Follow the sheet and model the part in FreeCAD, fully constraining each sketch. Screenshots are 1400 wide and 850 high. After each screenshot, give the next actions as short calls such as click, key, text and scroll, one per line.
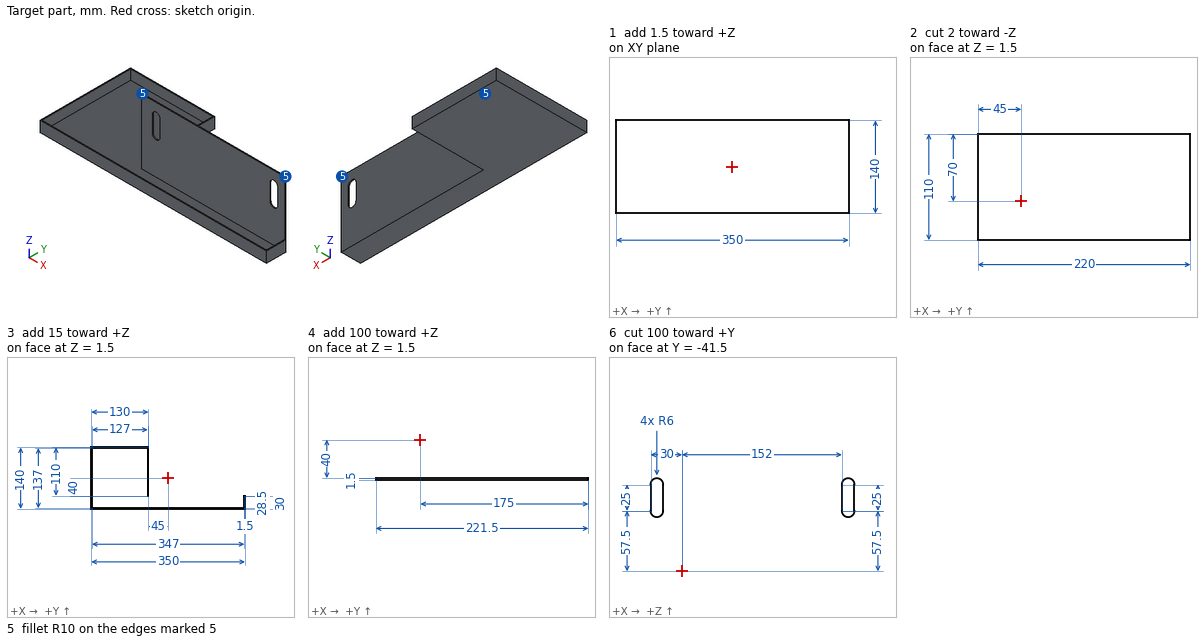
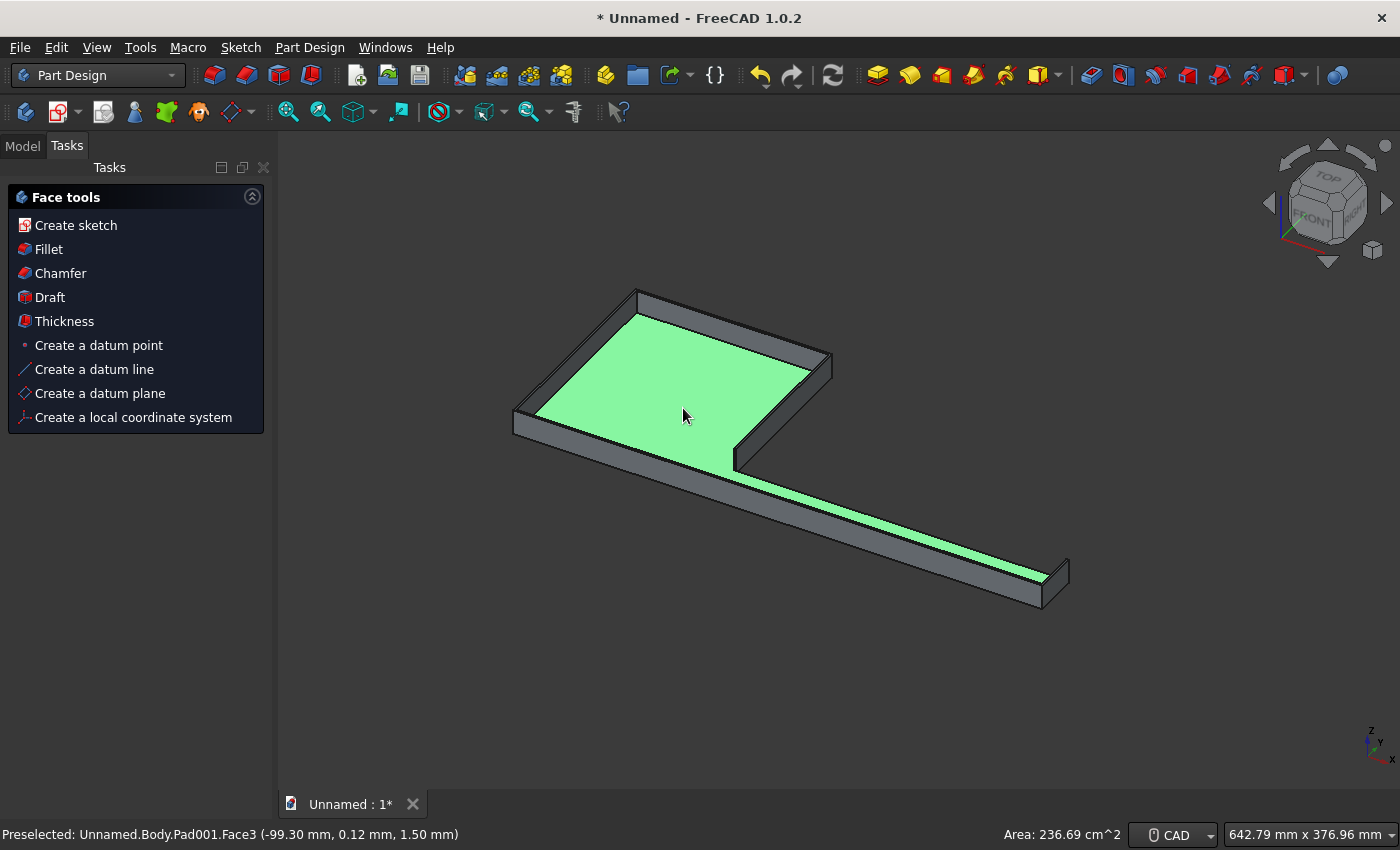
click(58, 112)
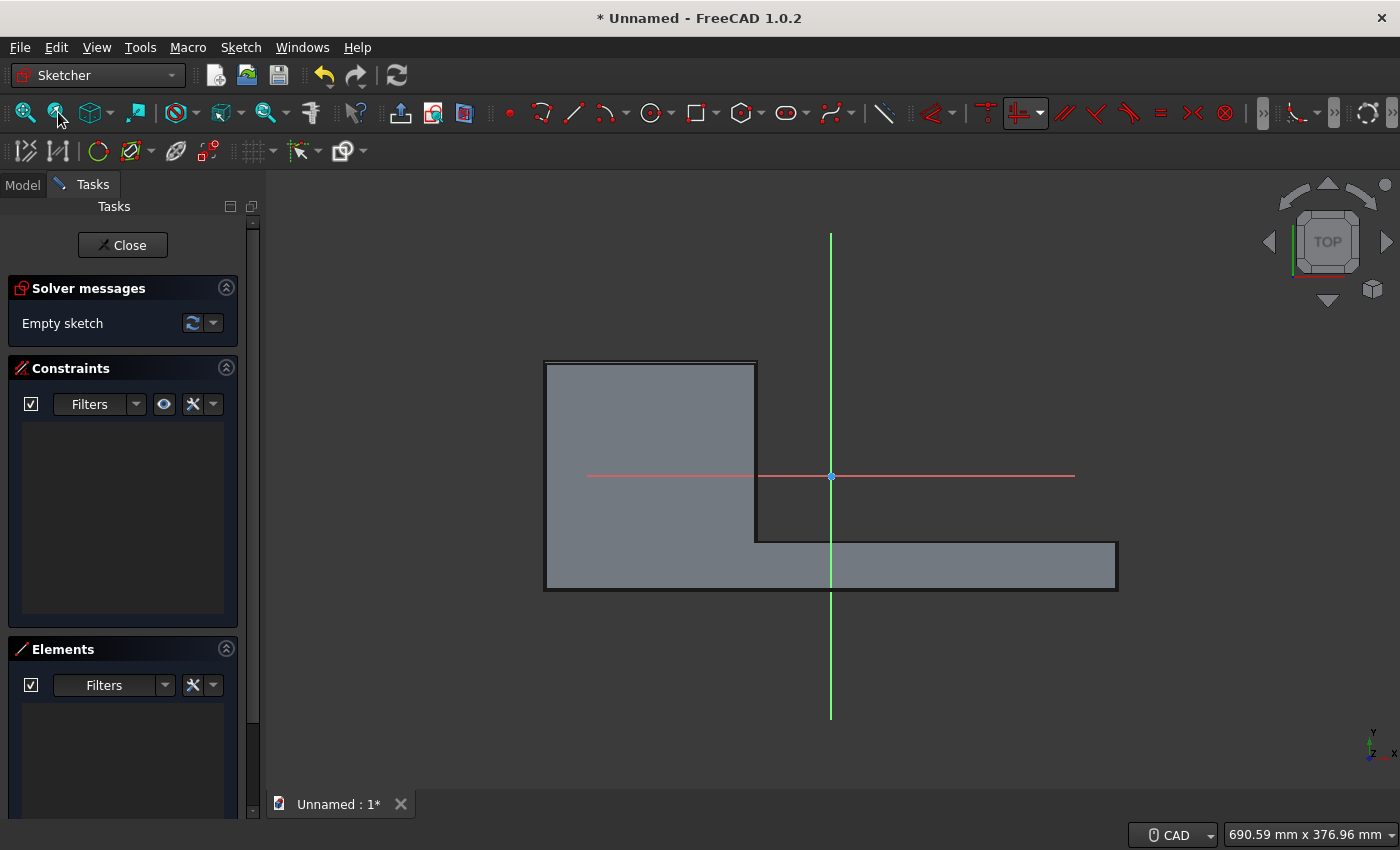
scroll(1146, 548, up, 3)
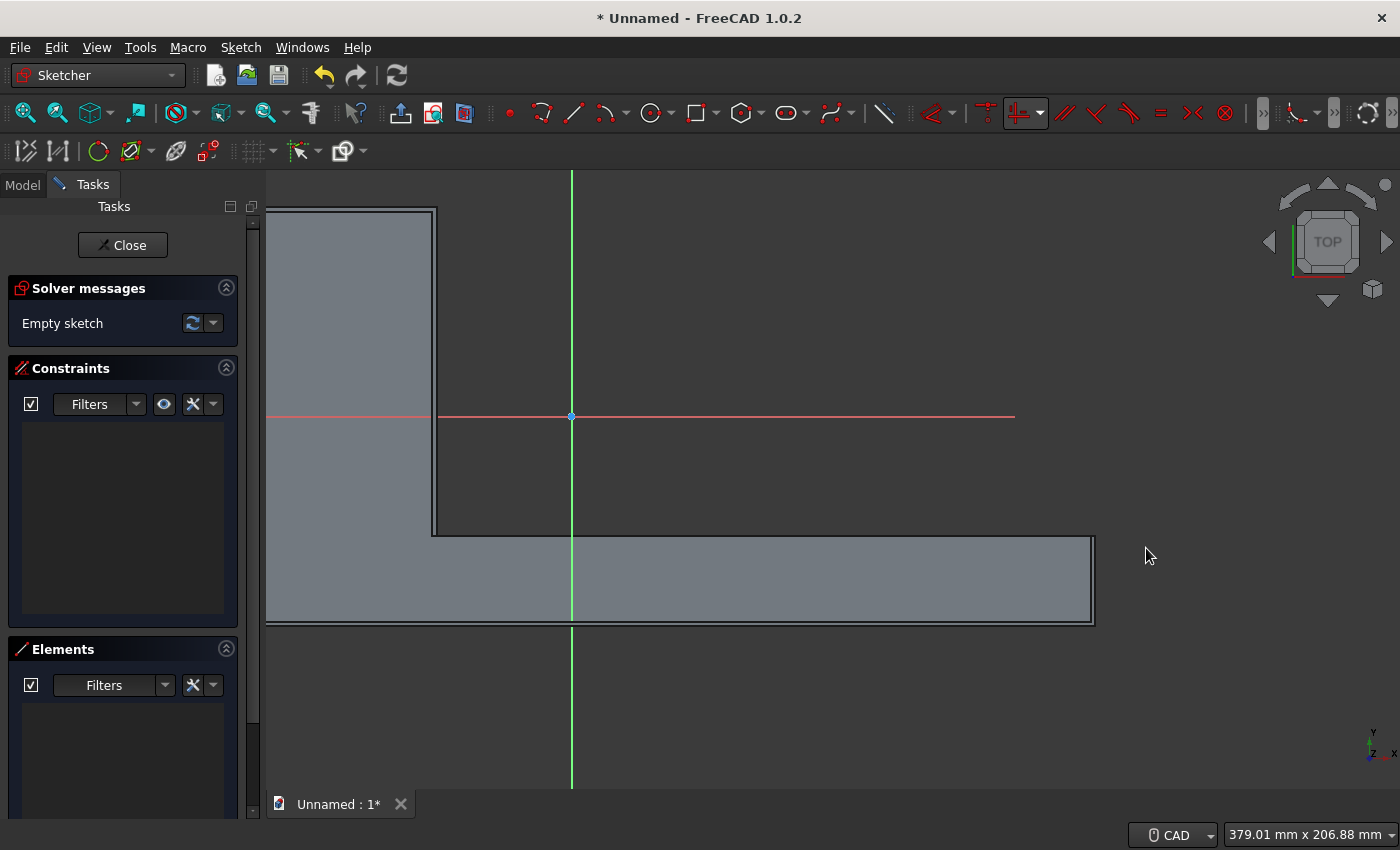
click(696, 114)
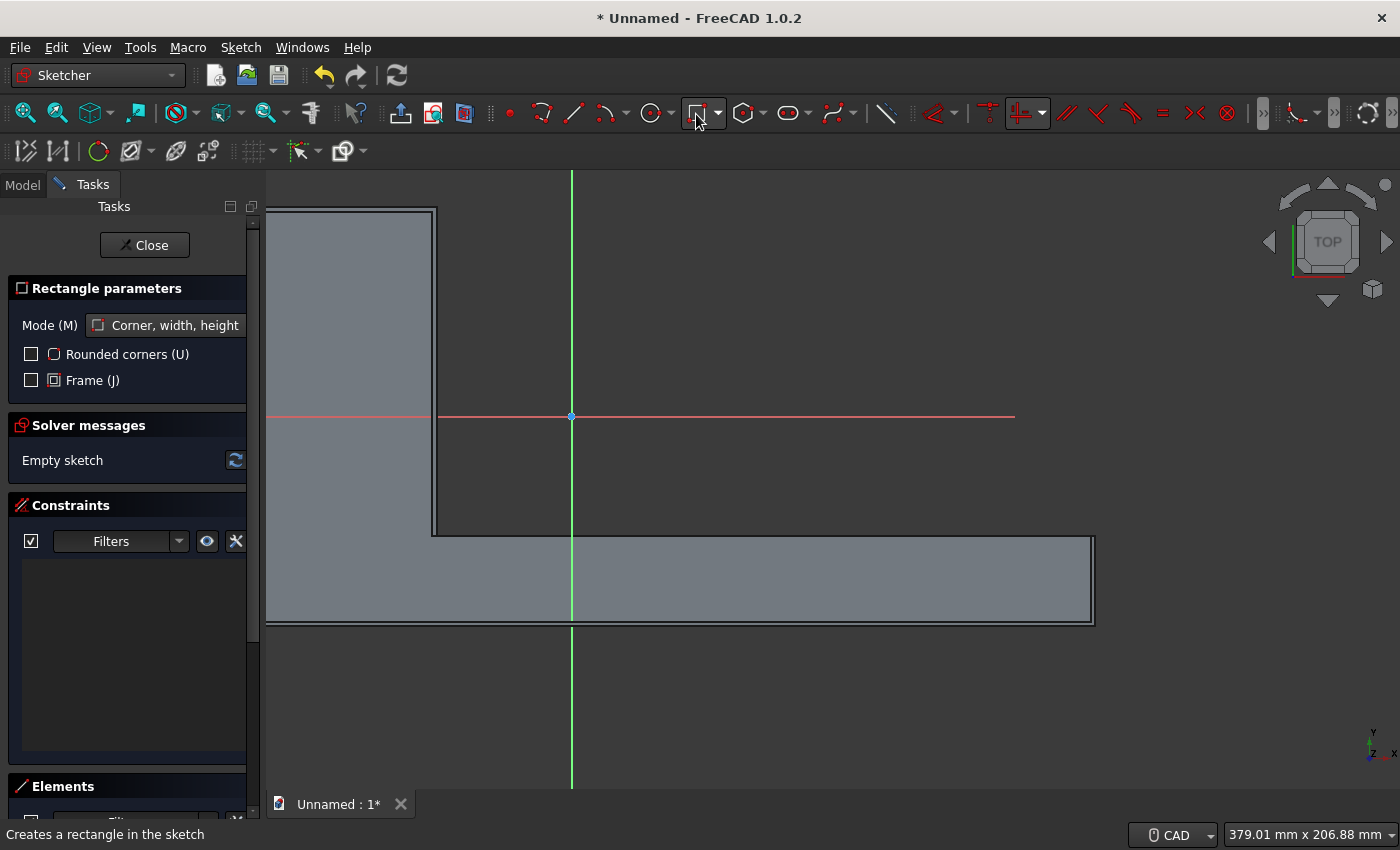
scroll(432, 536, up, 7)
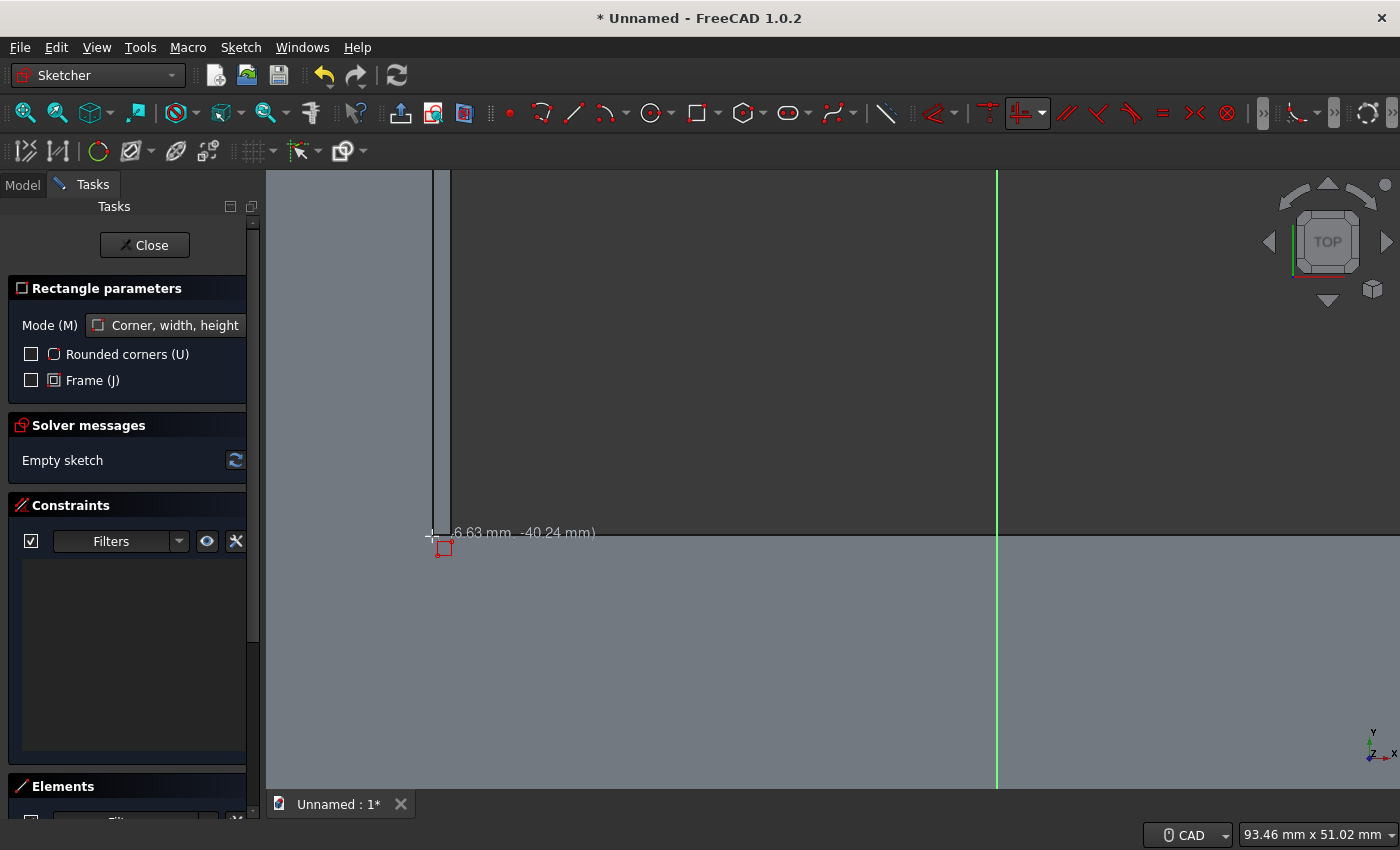
scroll(433, 538, down, 7)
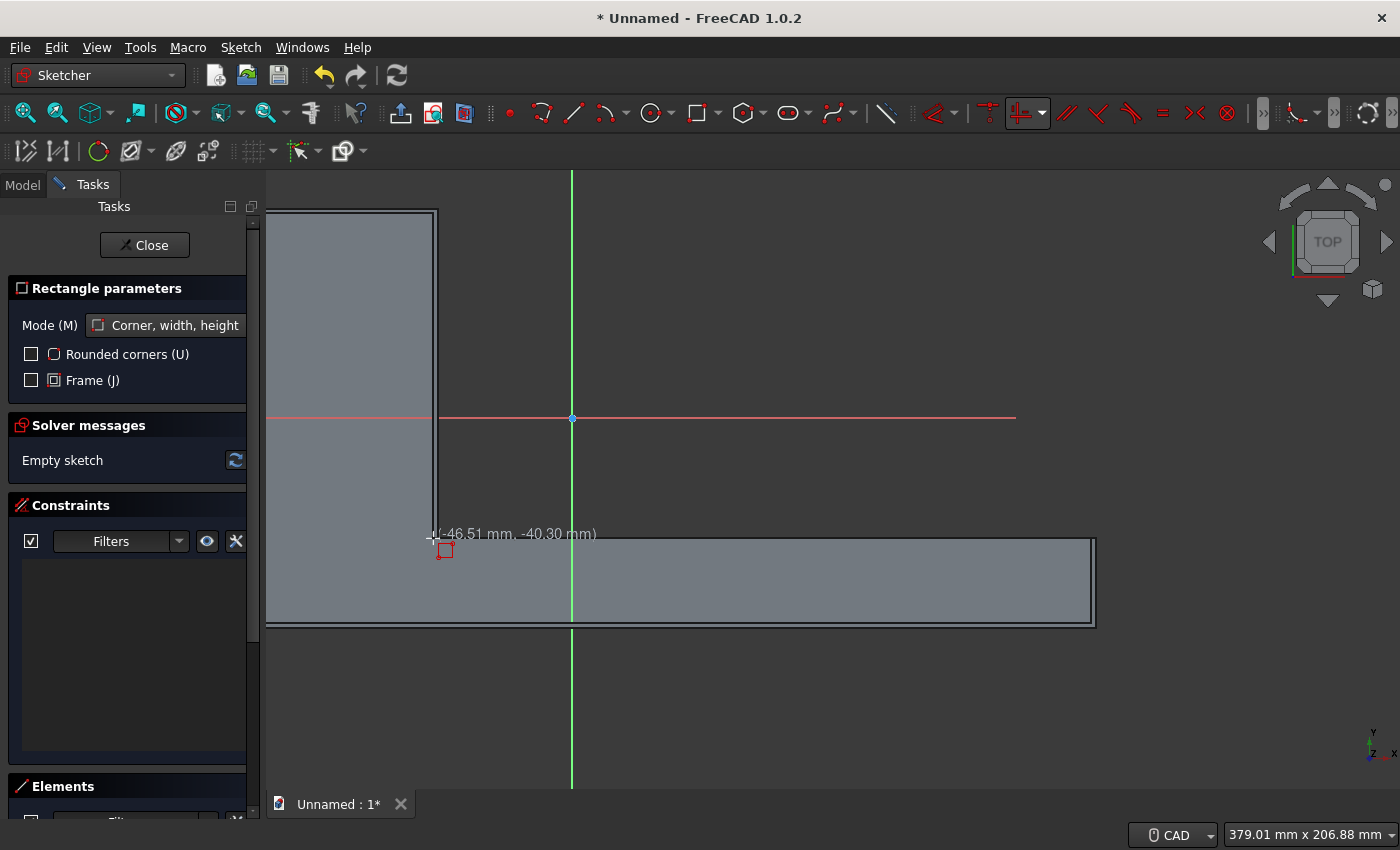
click(433, 538)
click(1096, 542)
key(Escape)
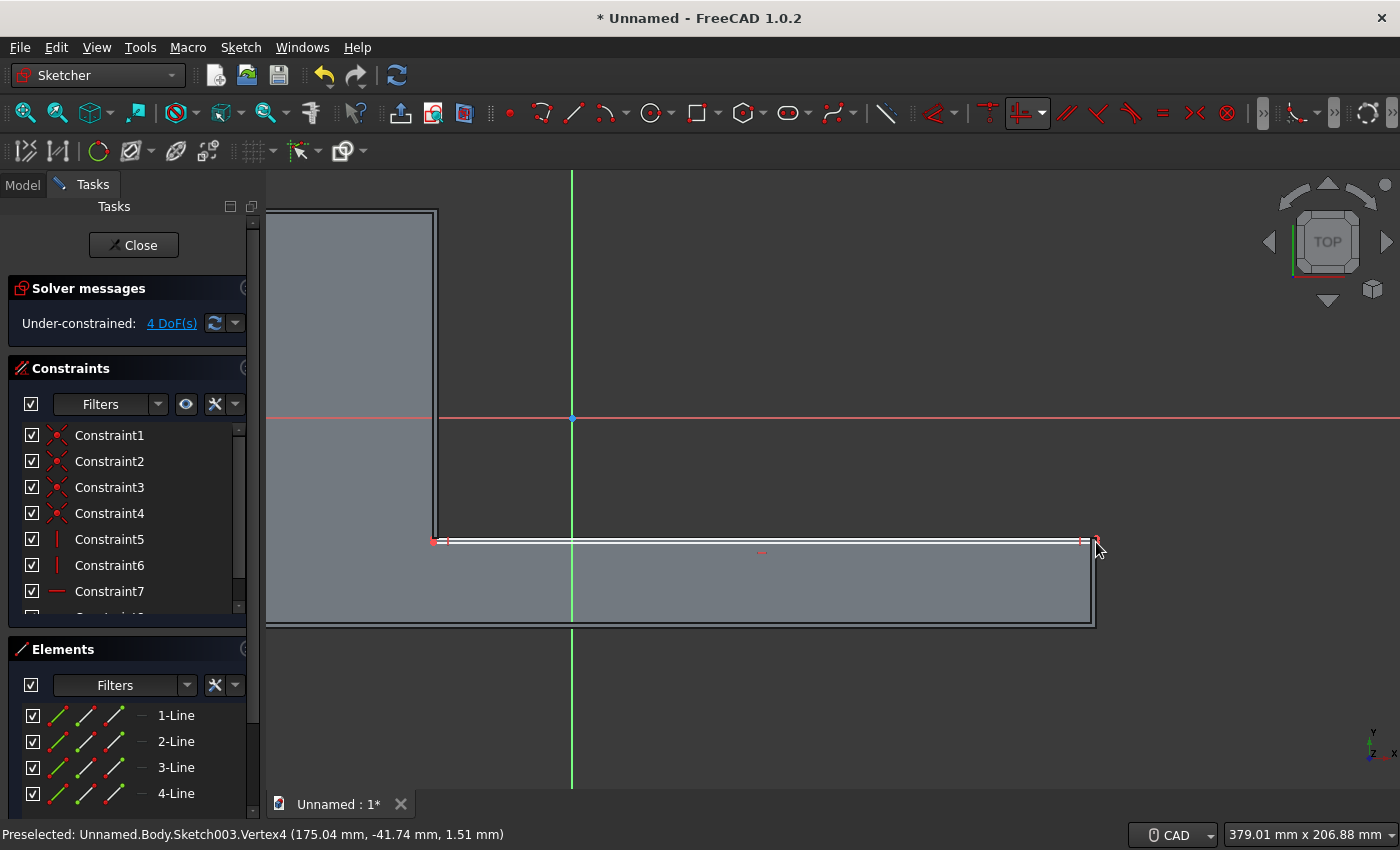
click(934, 114)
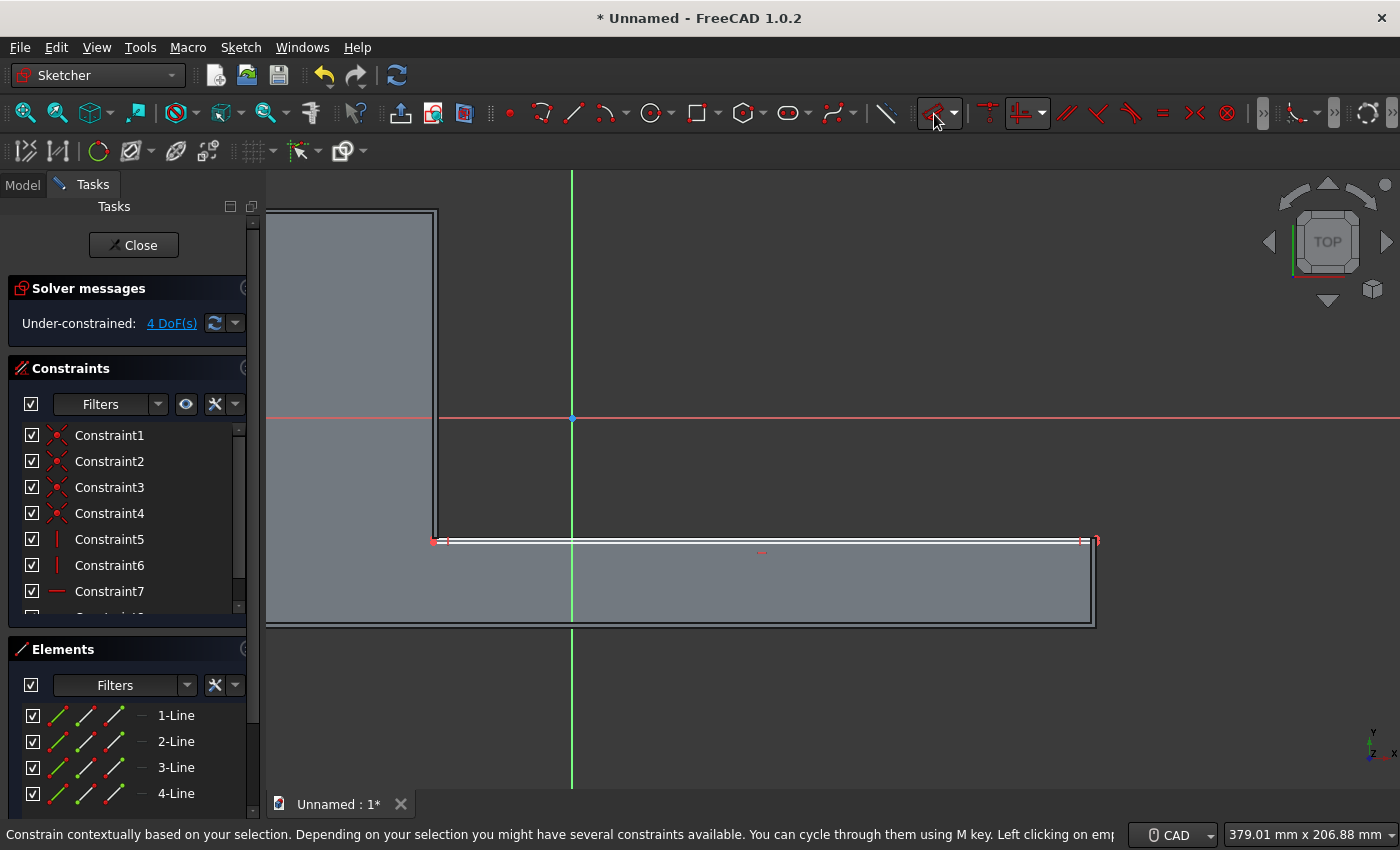
scroll(433, 541, up, 11)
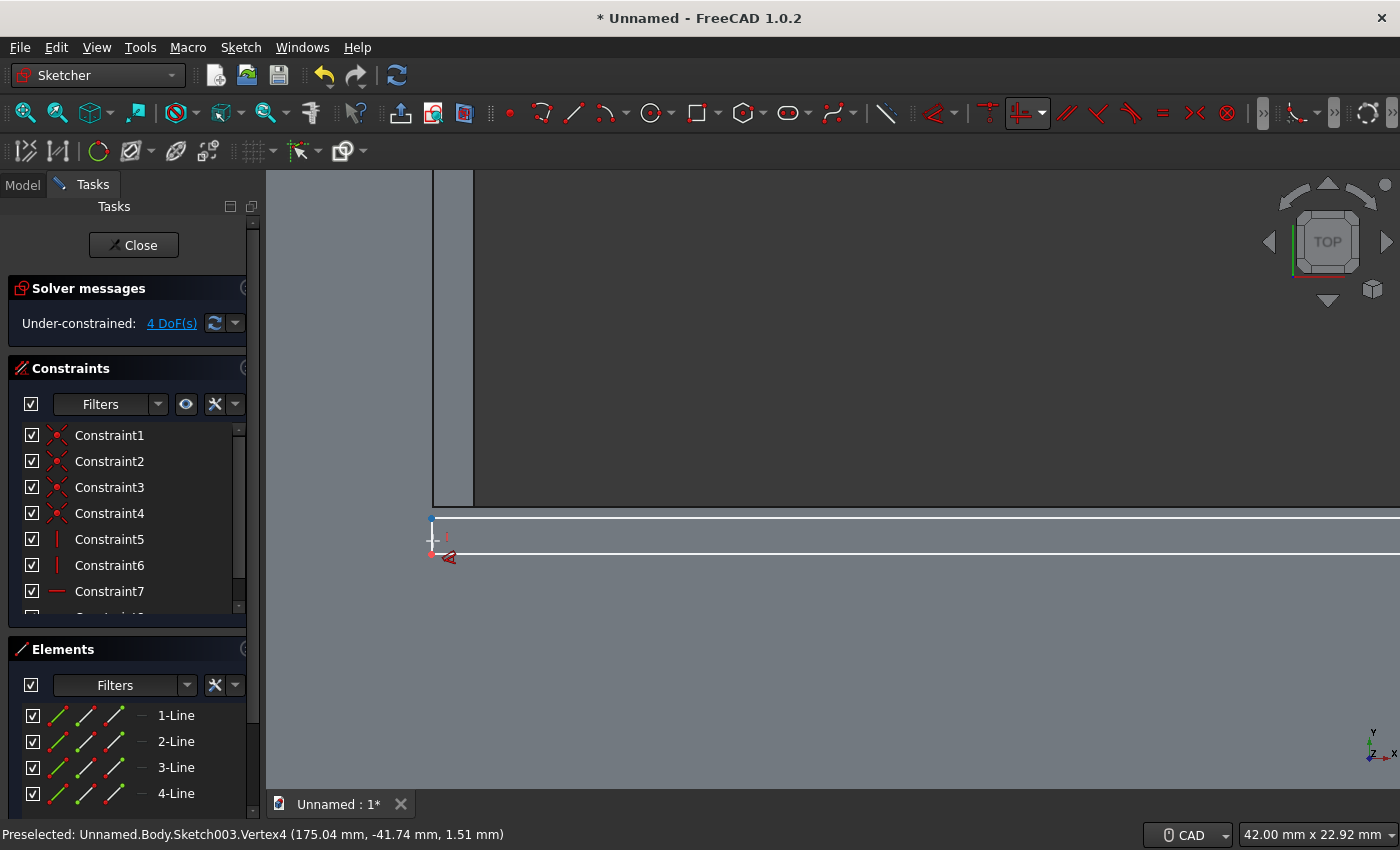
click(432, 536)
click(398, 536)